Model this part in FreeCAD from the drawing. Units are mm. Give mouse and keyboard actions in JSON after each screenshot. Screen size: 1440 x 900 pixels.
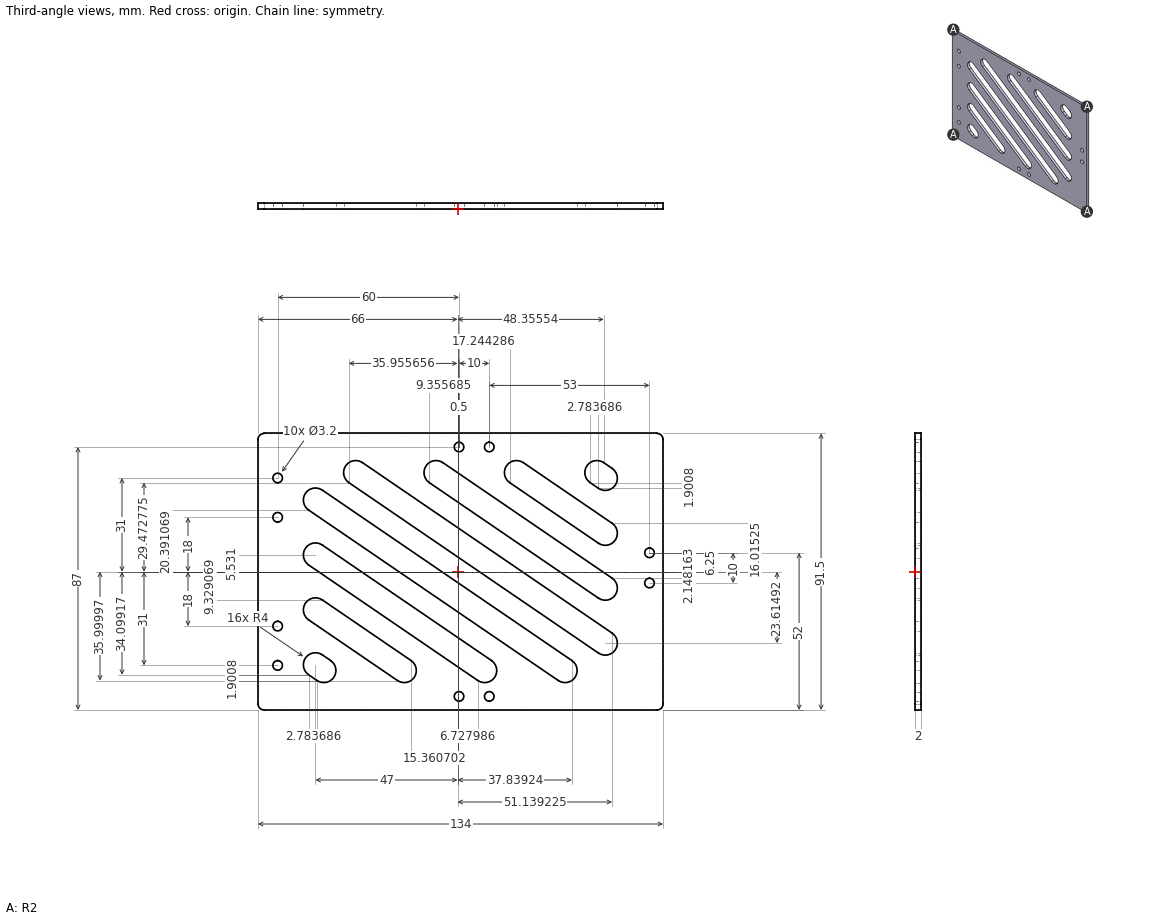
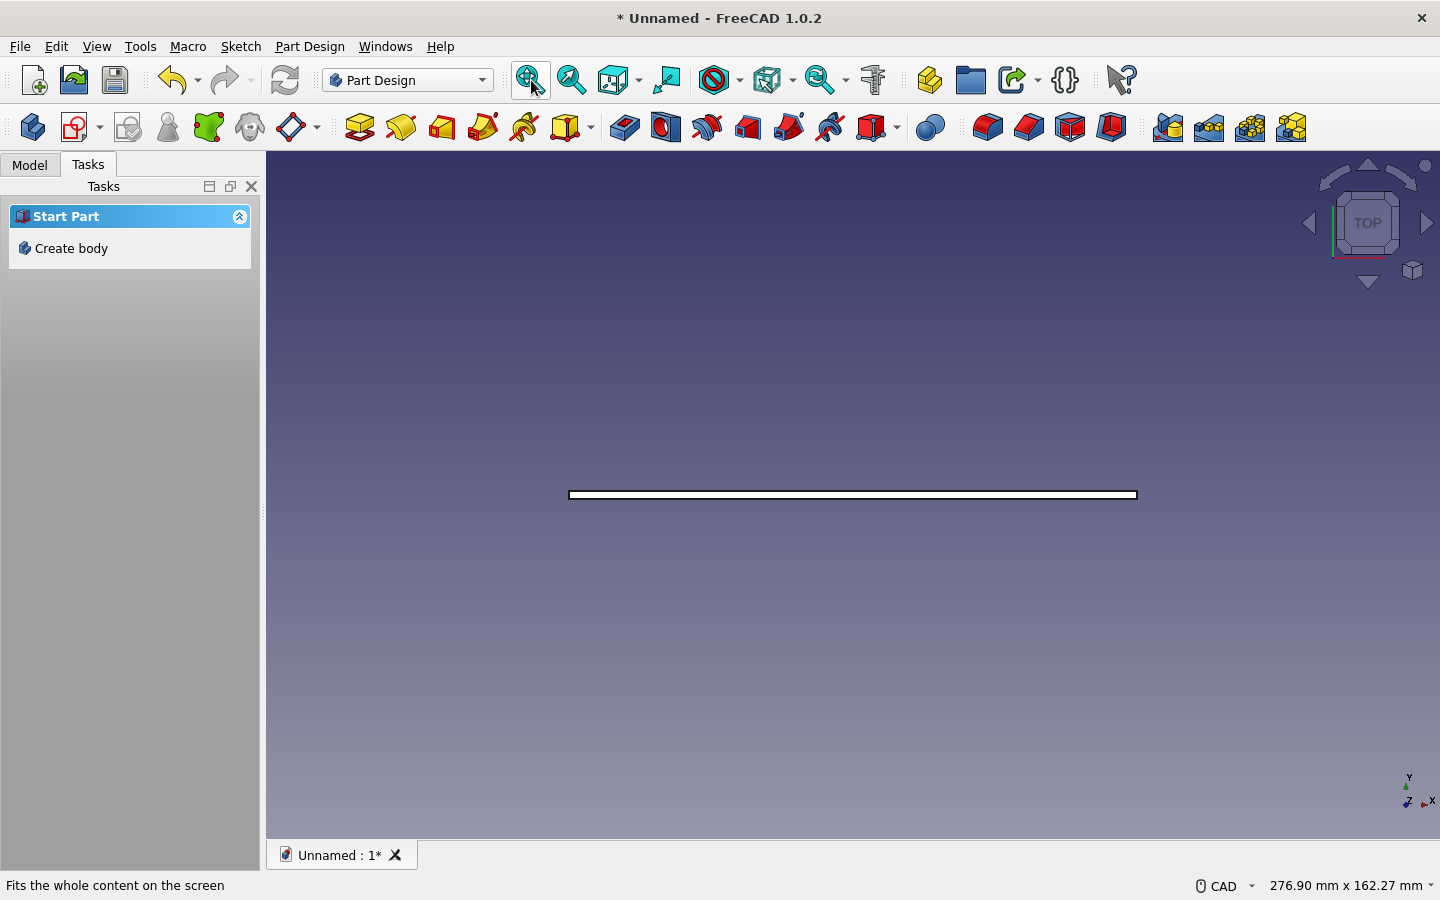
{"action": "left_click", "coordinate": [1137, 496]}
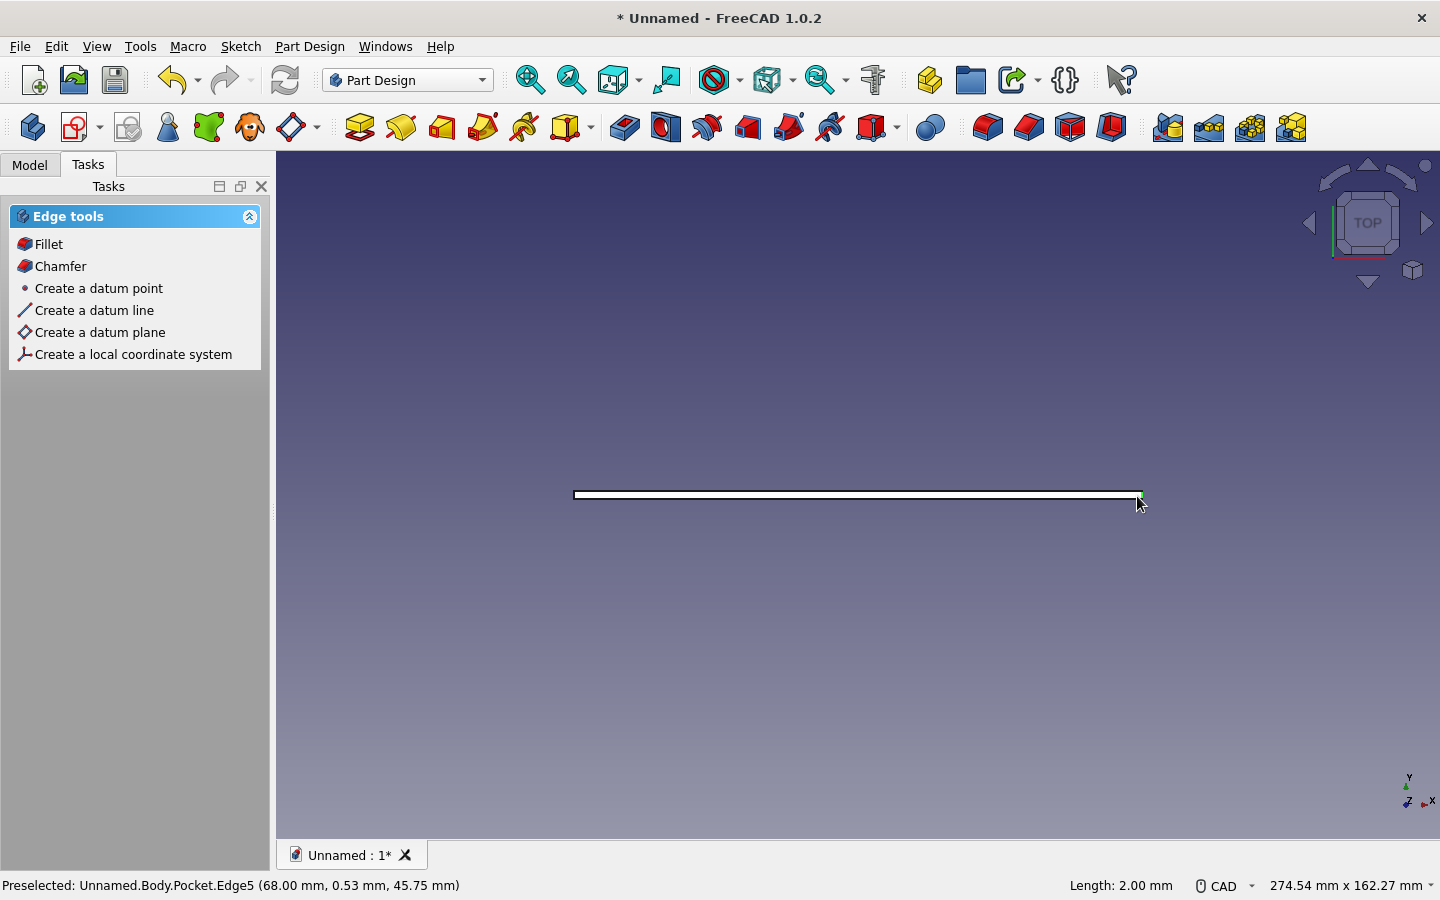
{"action": "left_click", "coordinate": [574, 496], "text": "ctrl"}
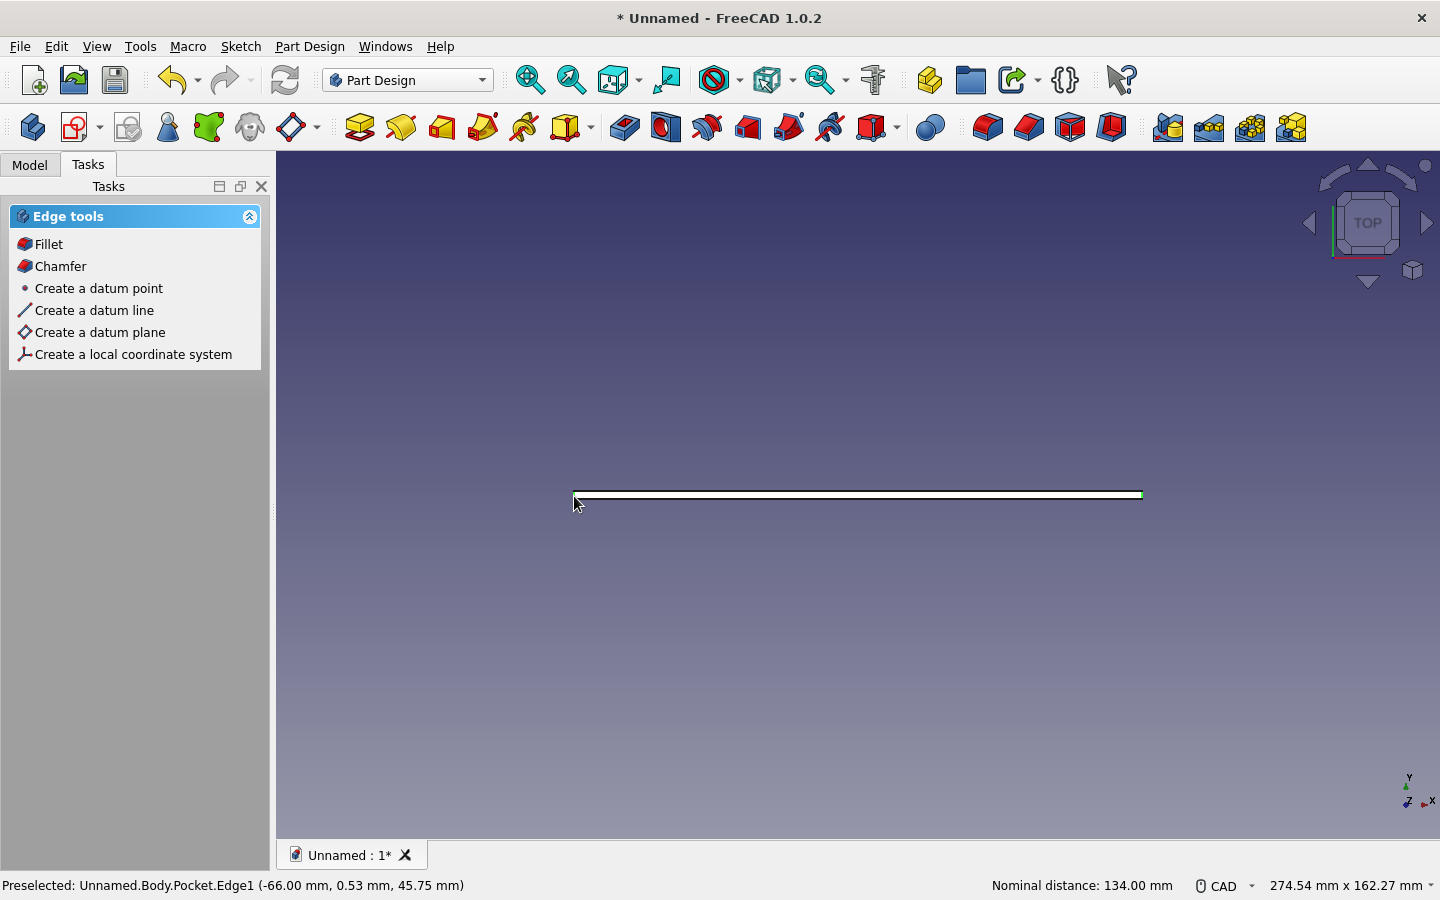
{"action": "scroll", "coordinate": [574, 494], "scroll_direction": "up", "scroll_amount": 8}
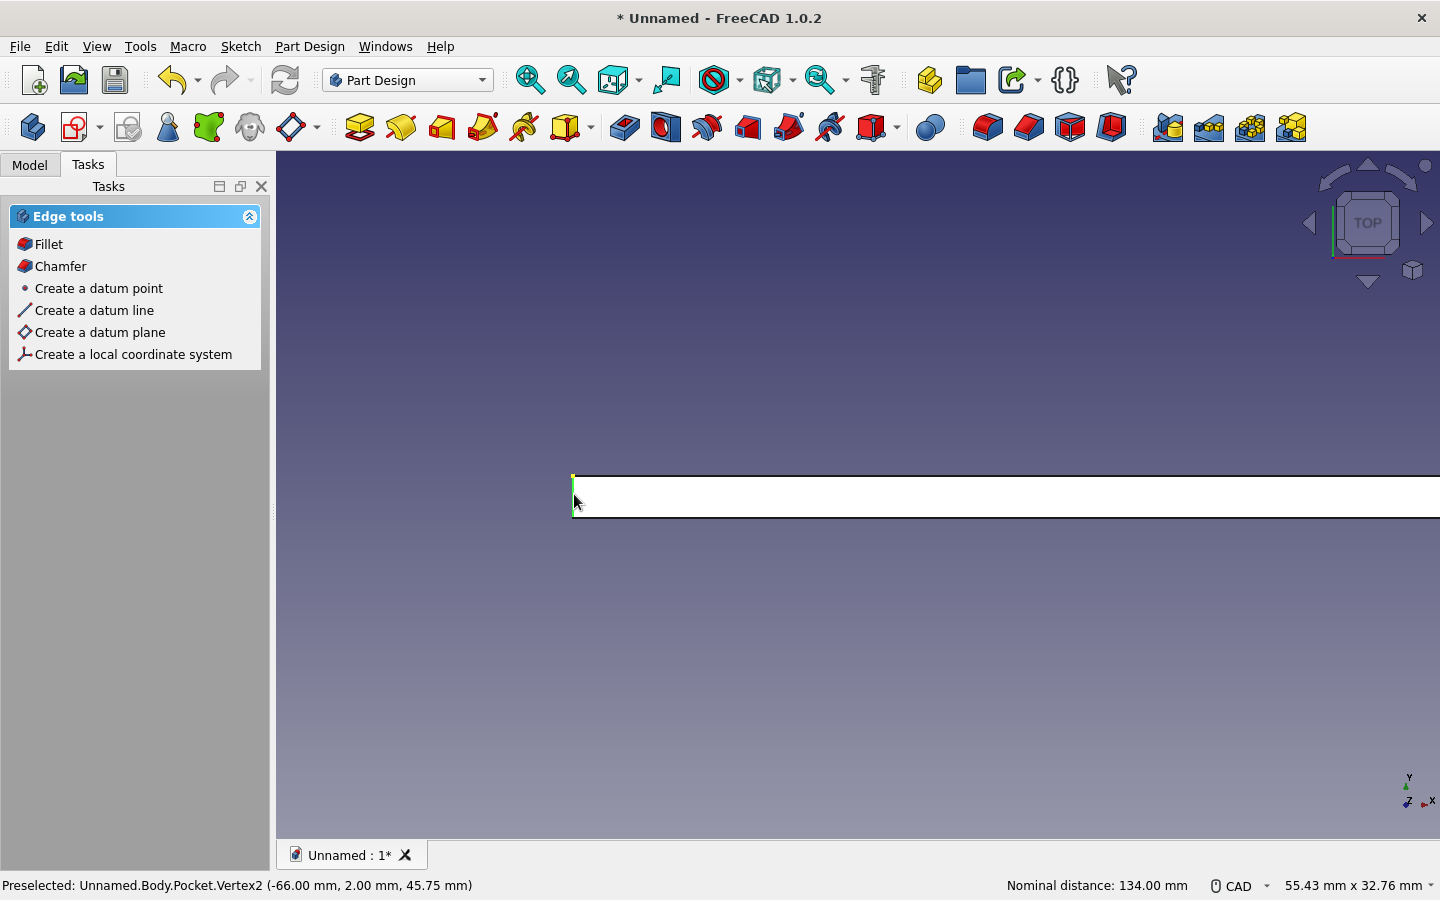
{"action": "left_click", "coordinate": [531, 80]}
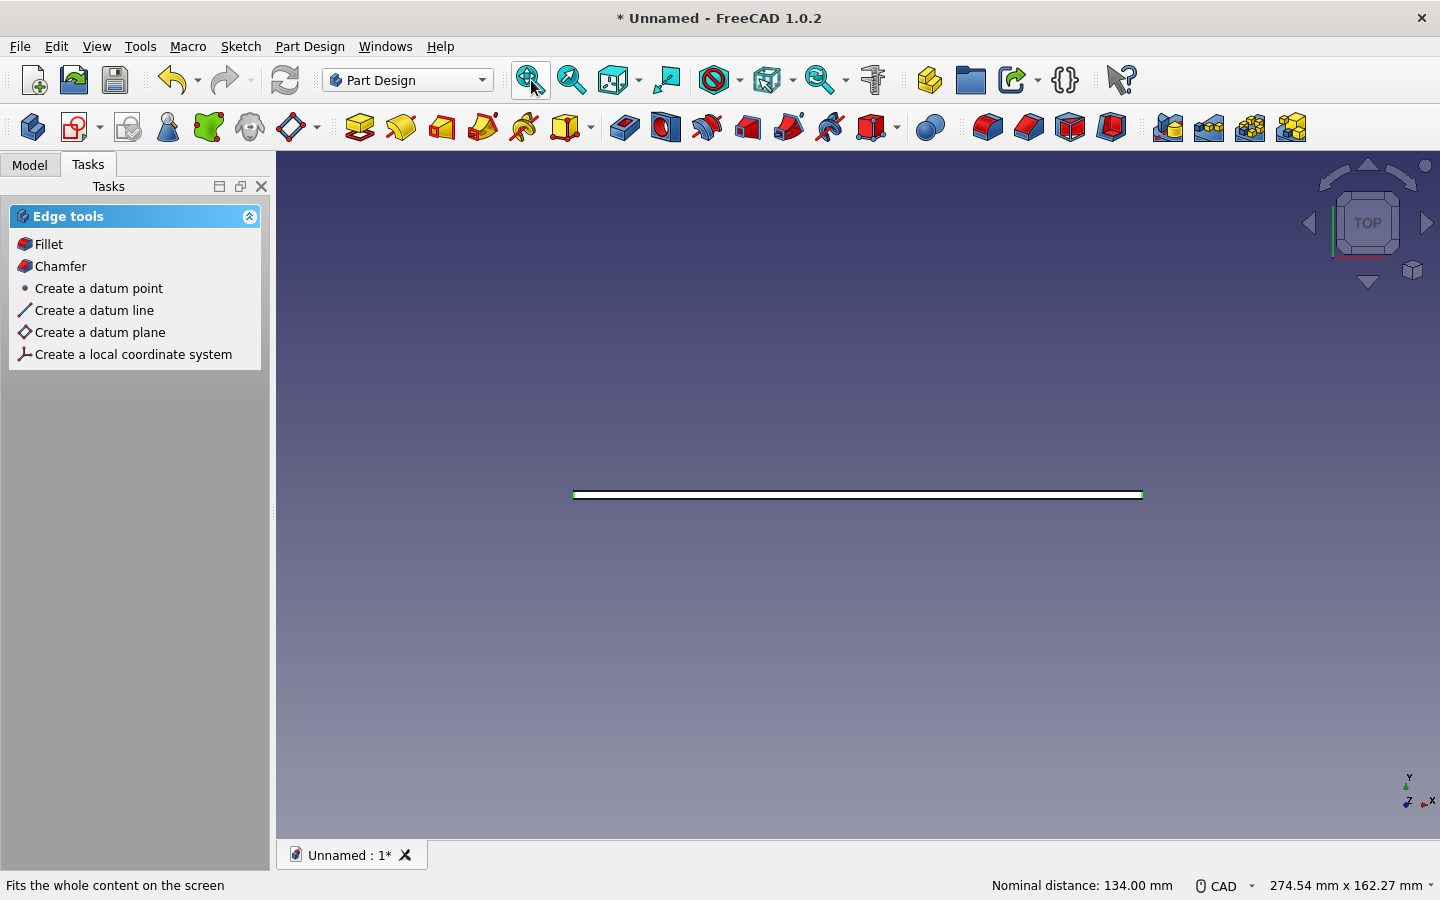
{"action": "key", "text": "1"}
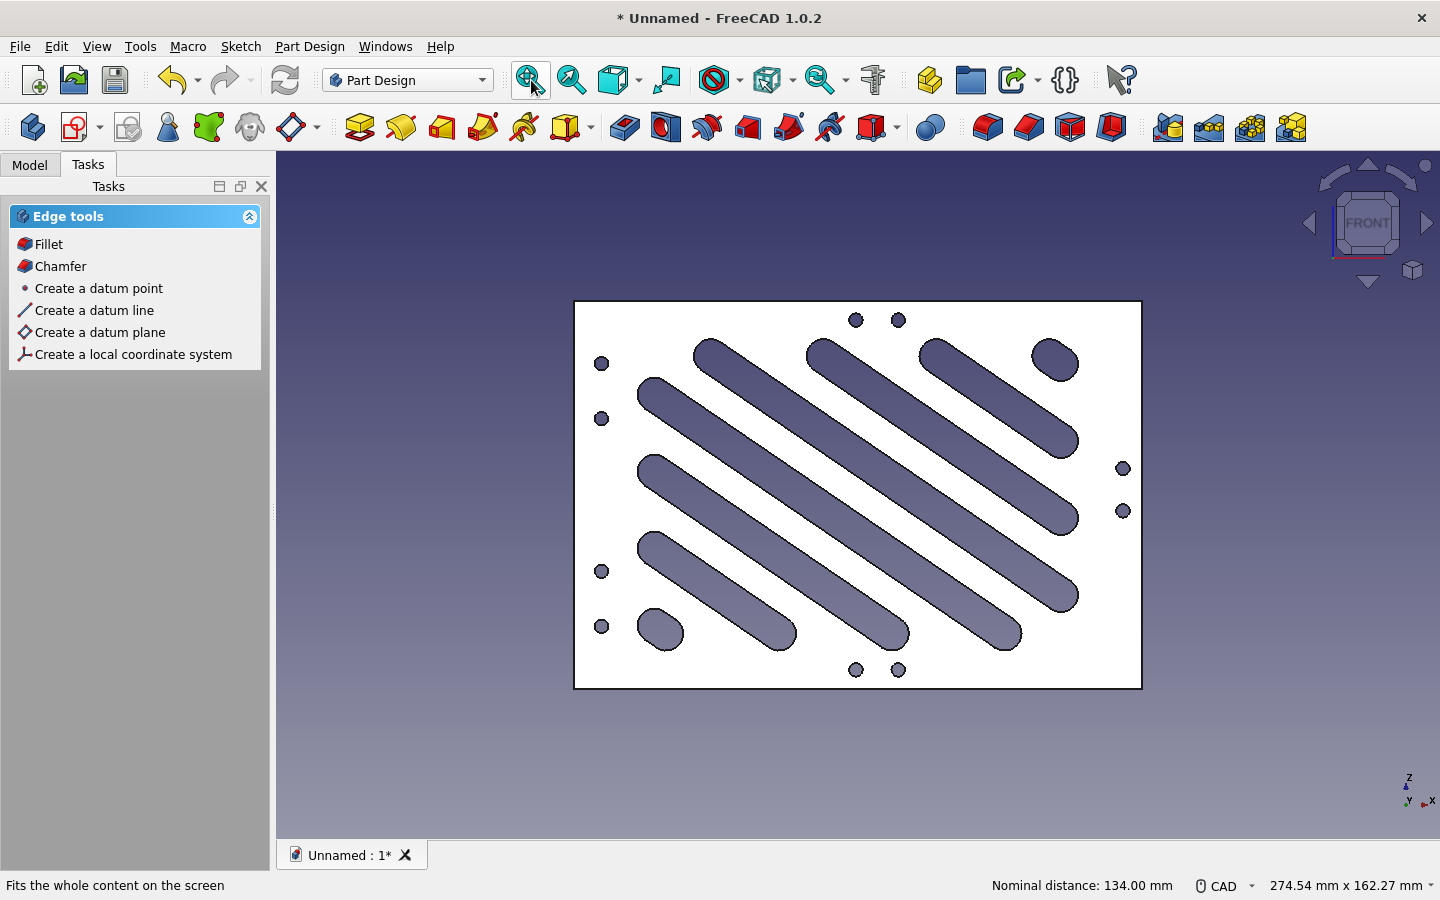
{"action": "scroll", "coordinate": [574, 688], "scroll_direction": "up", "scroll_amount": 8}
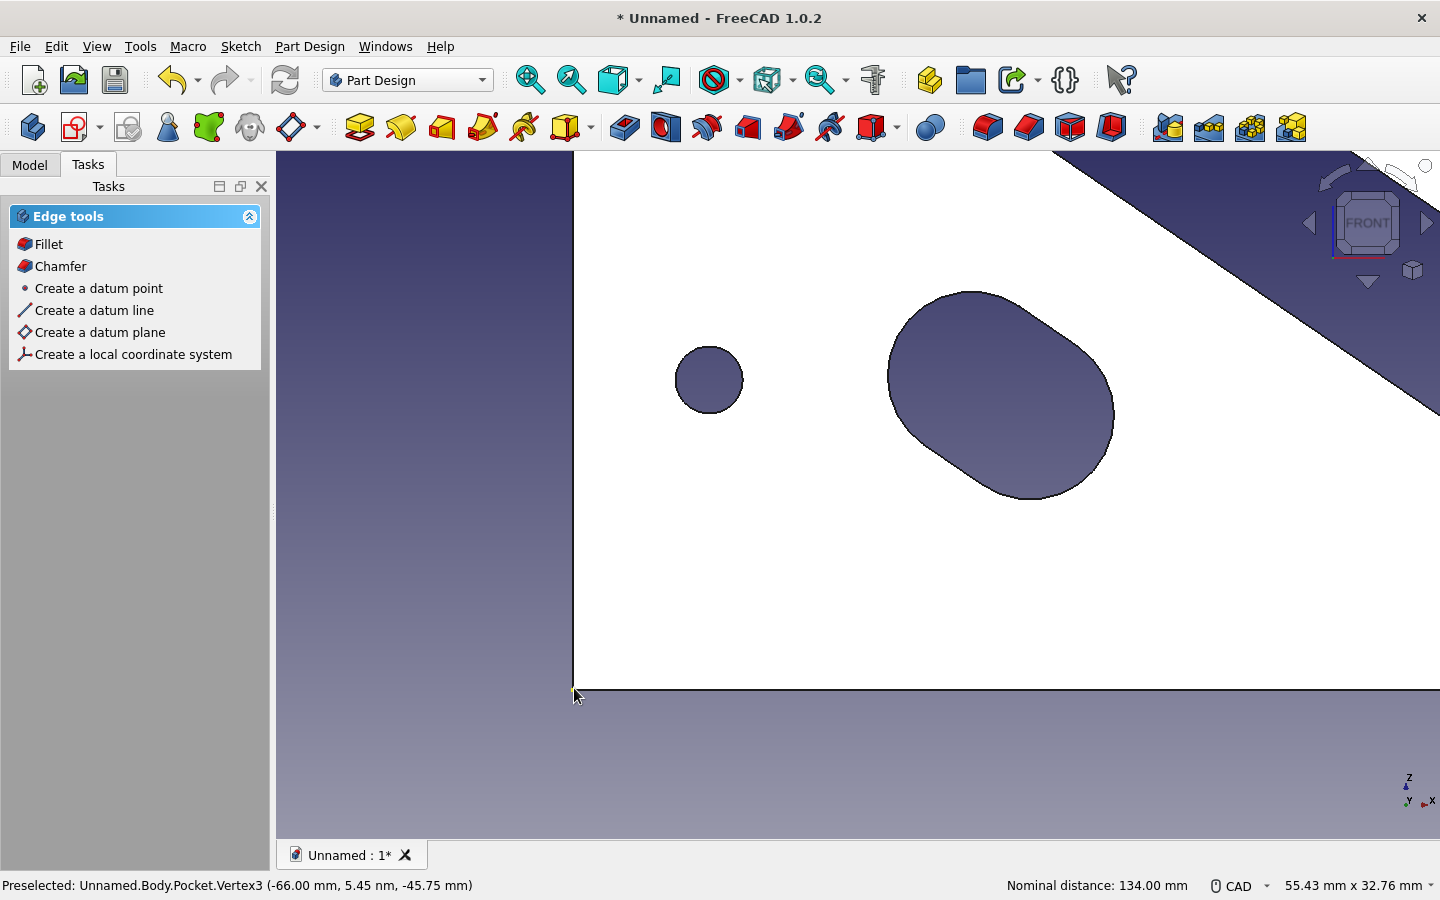
{"action": "left_click", "coordinate": [531, 80]}